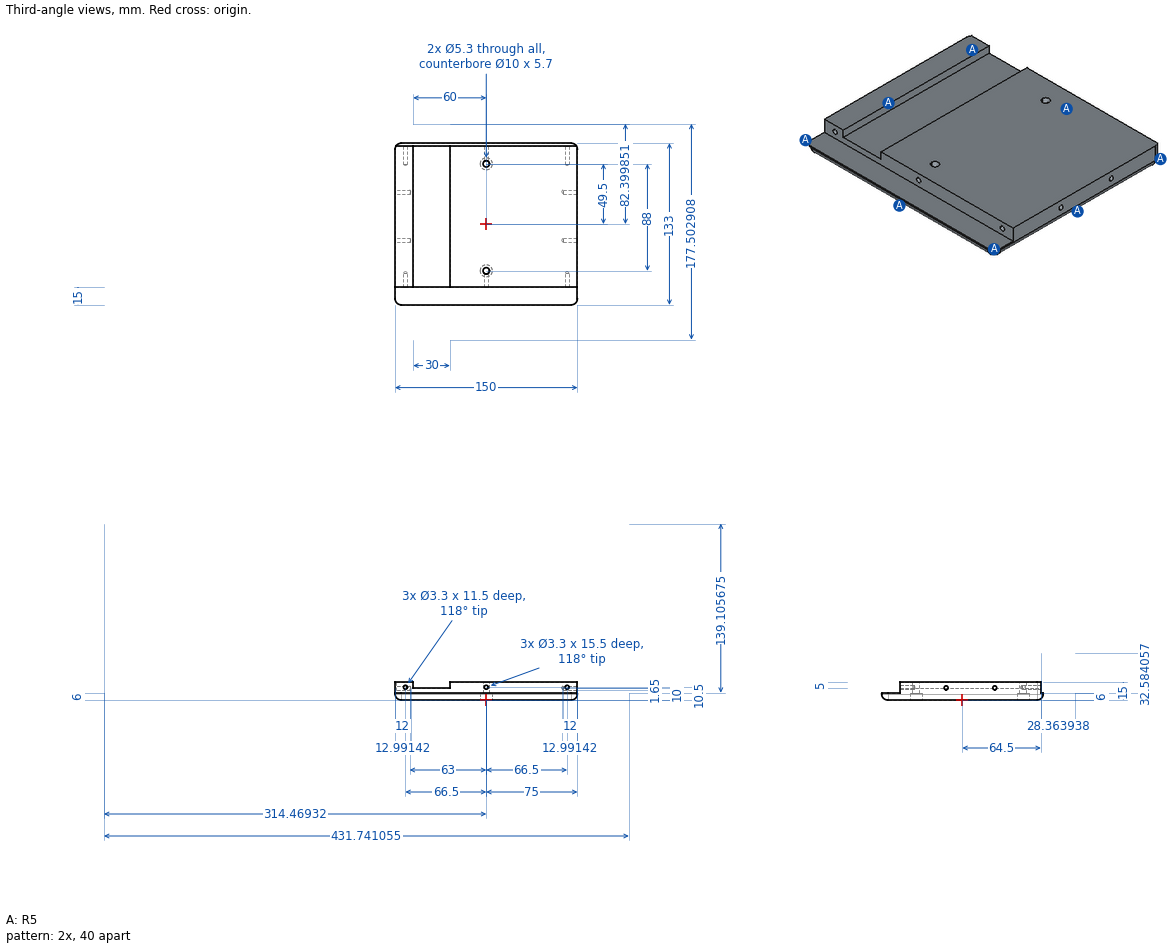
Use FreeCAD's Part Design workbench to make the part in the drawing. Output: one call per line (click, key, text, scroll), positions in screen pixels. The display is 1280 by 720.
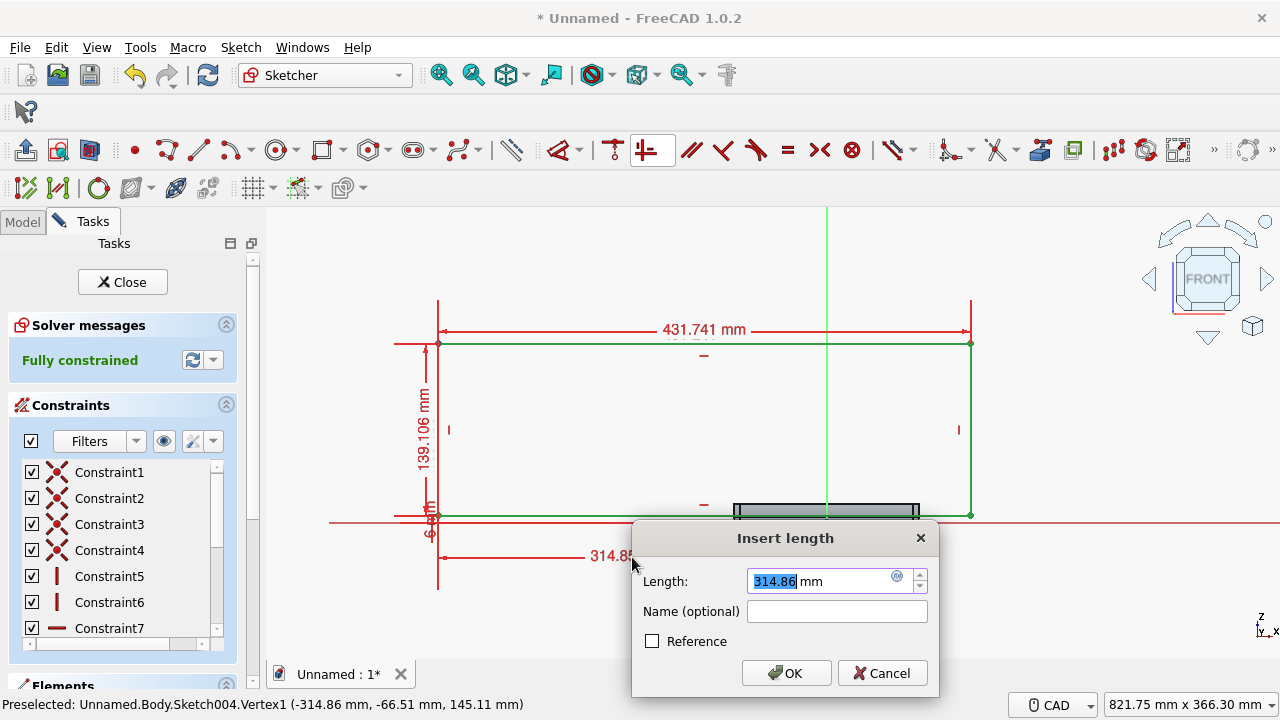
text(314.46932)
key(Return)
key(Escape)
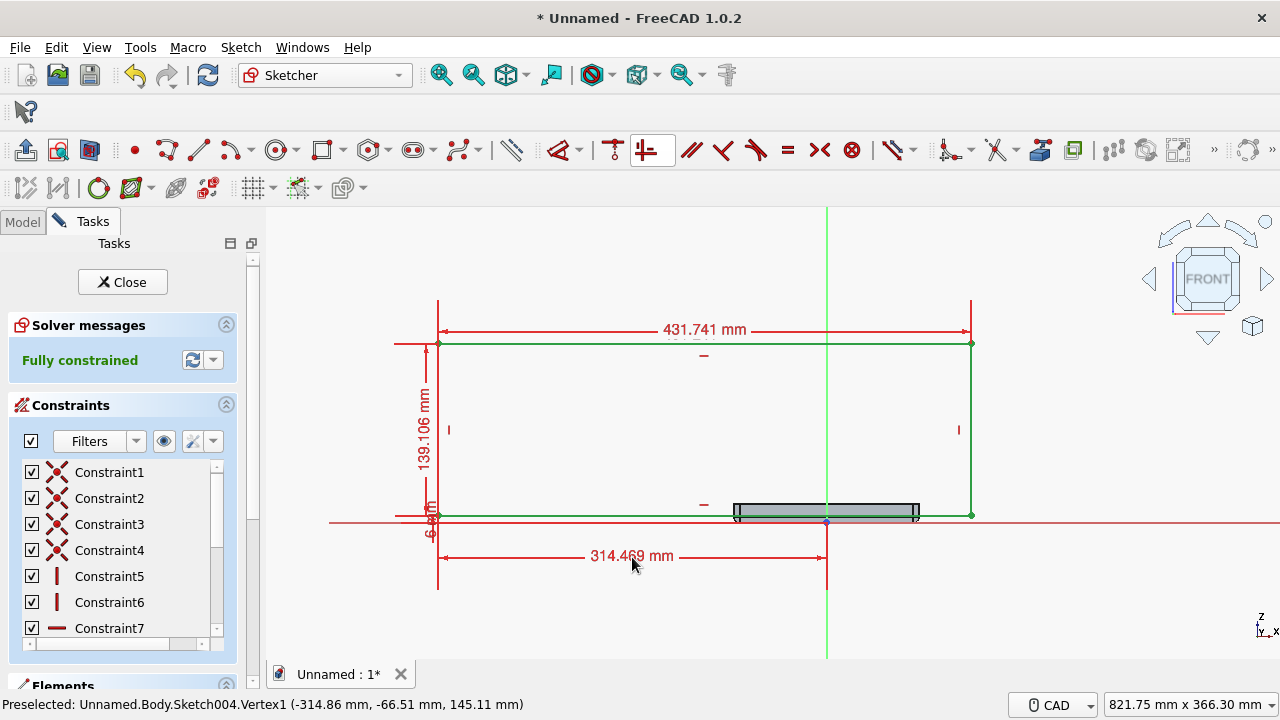
click(123, 282)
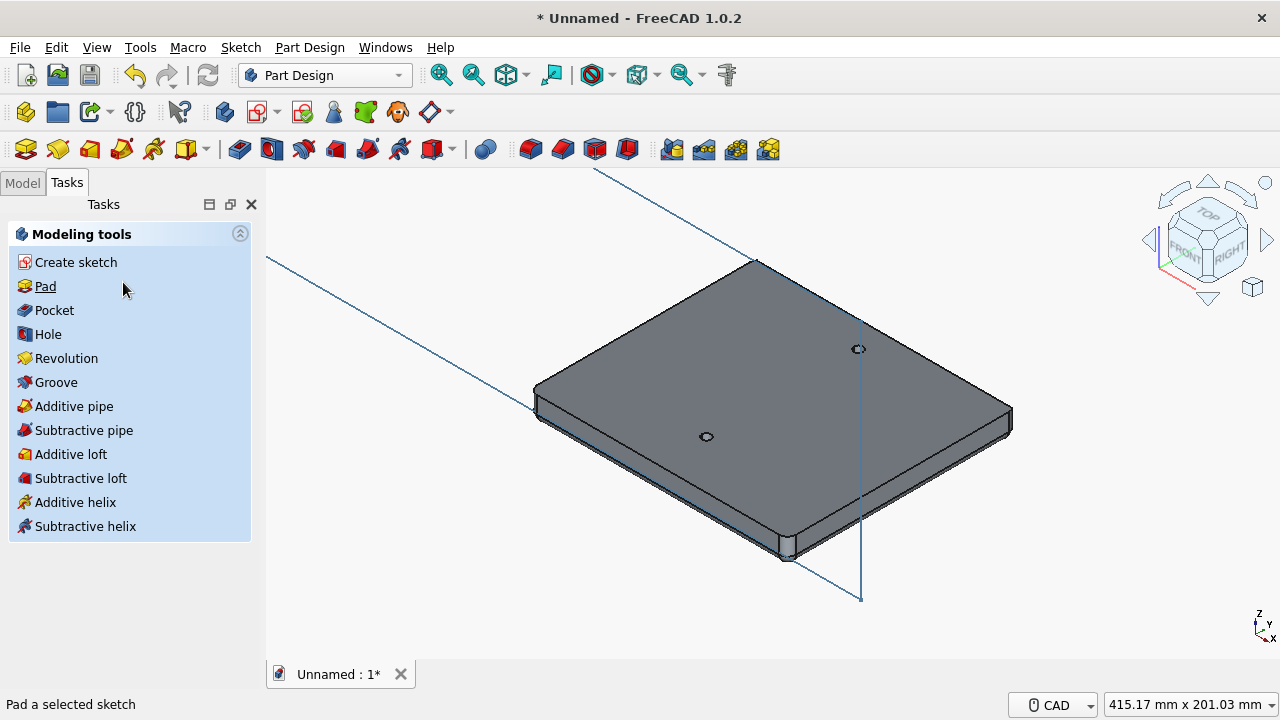
click(240, 150)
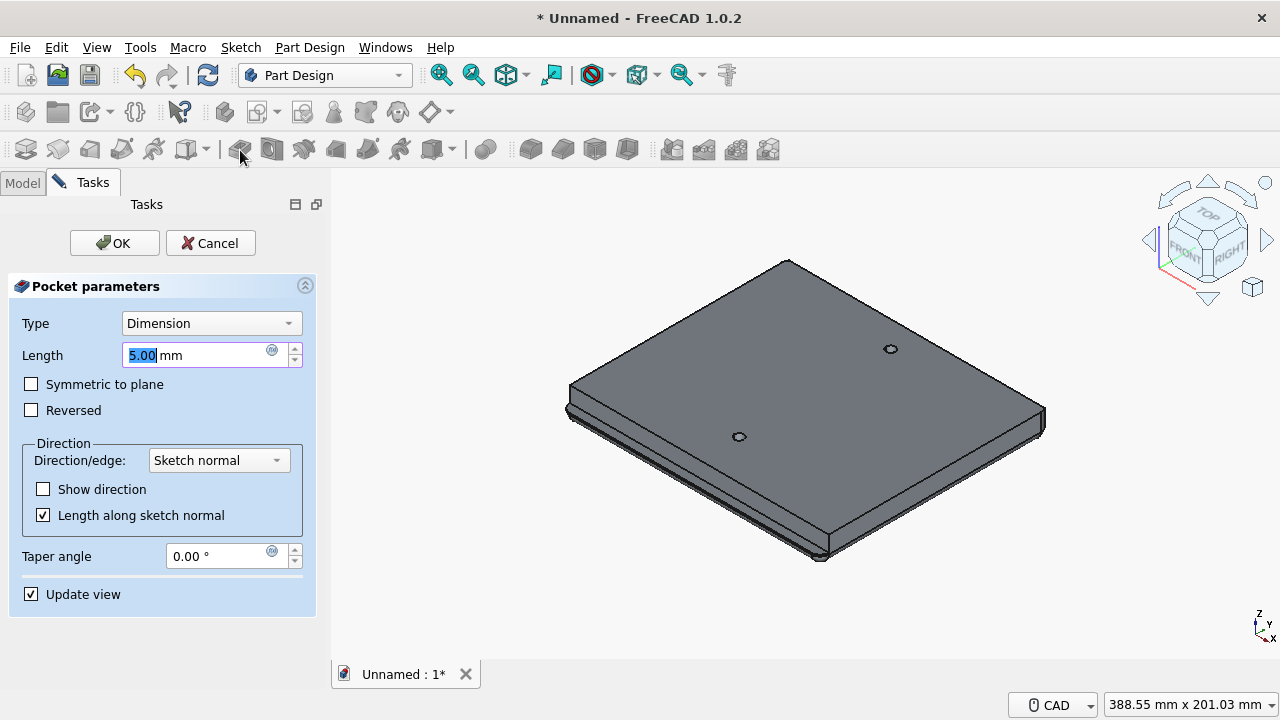
text(15)
key(Tab)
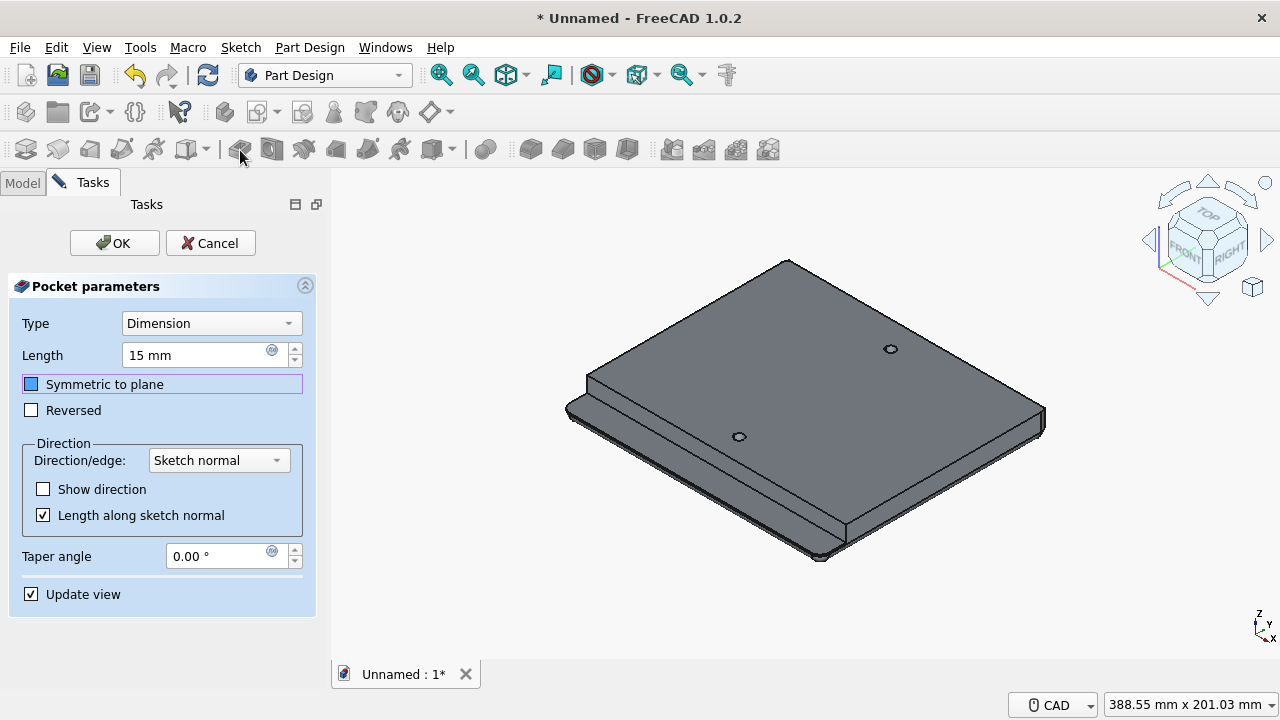
click(115, 243)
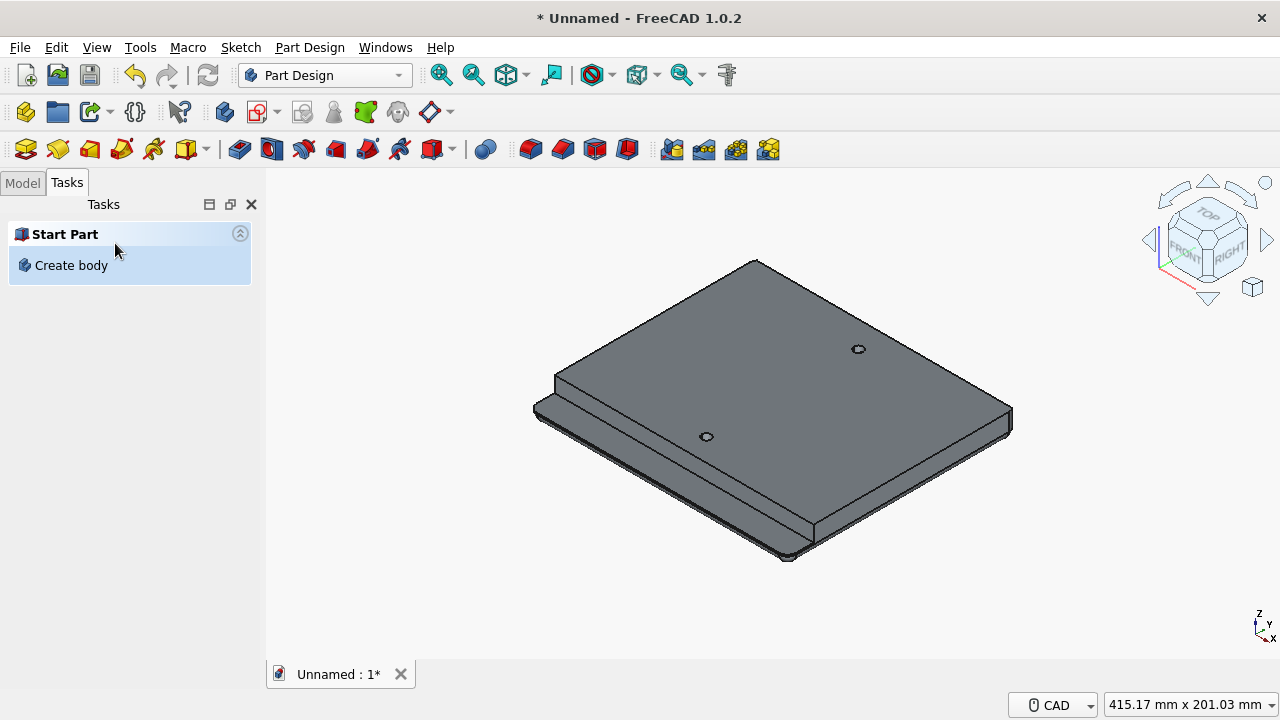
click(821, 412)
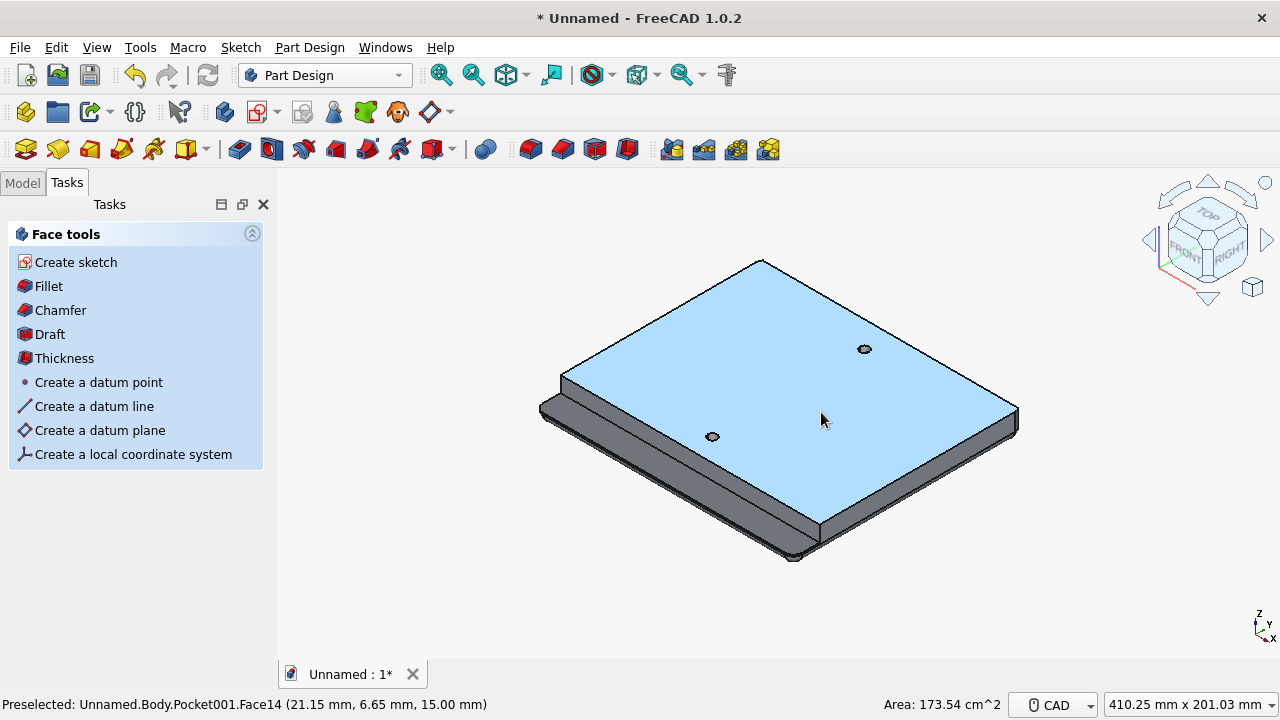
click(258, 112)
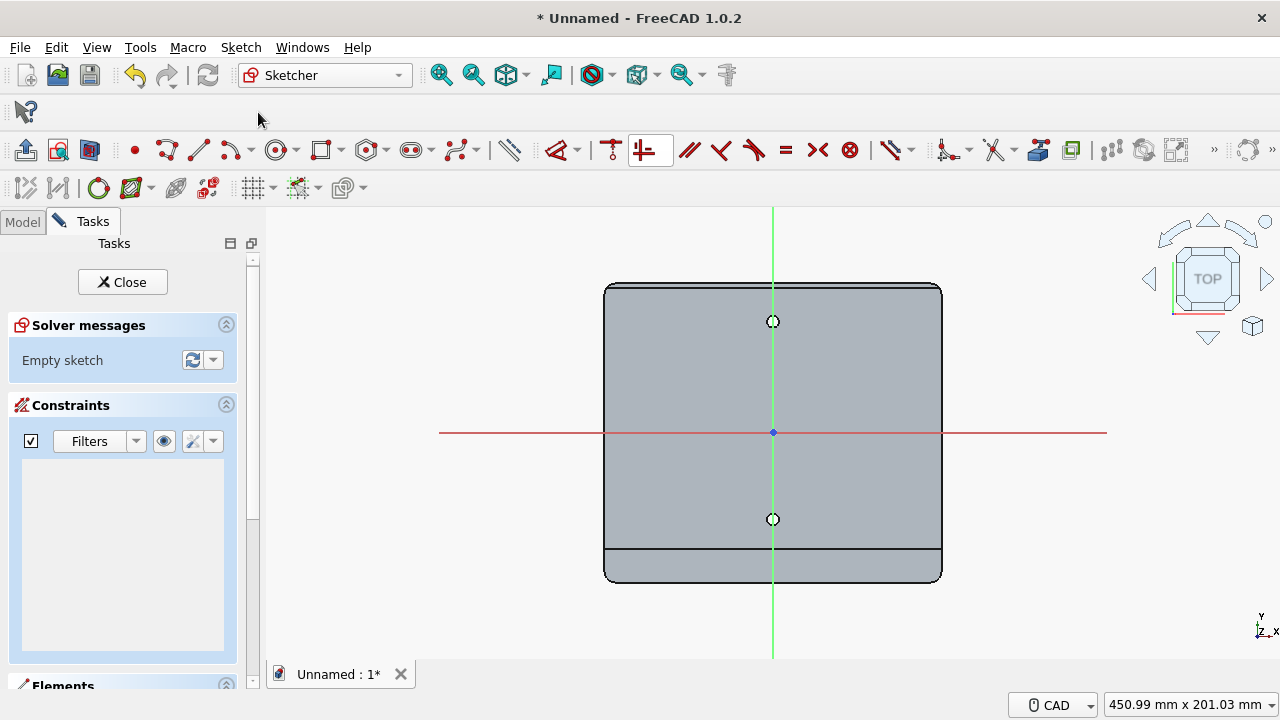
scroll(702, 404, down, 2)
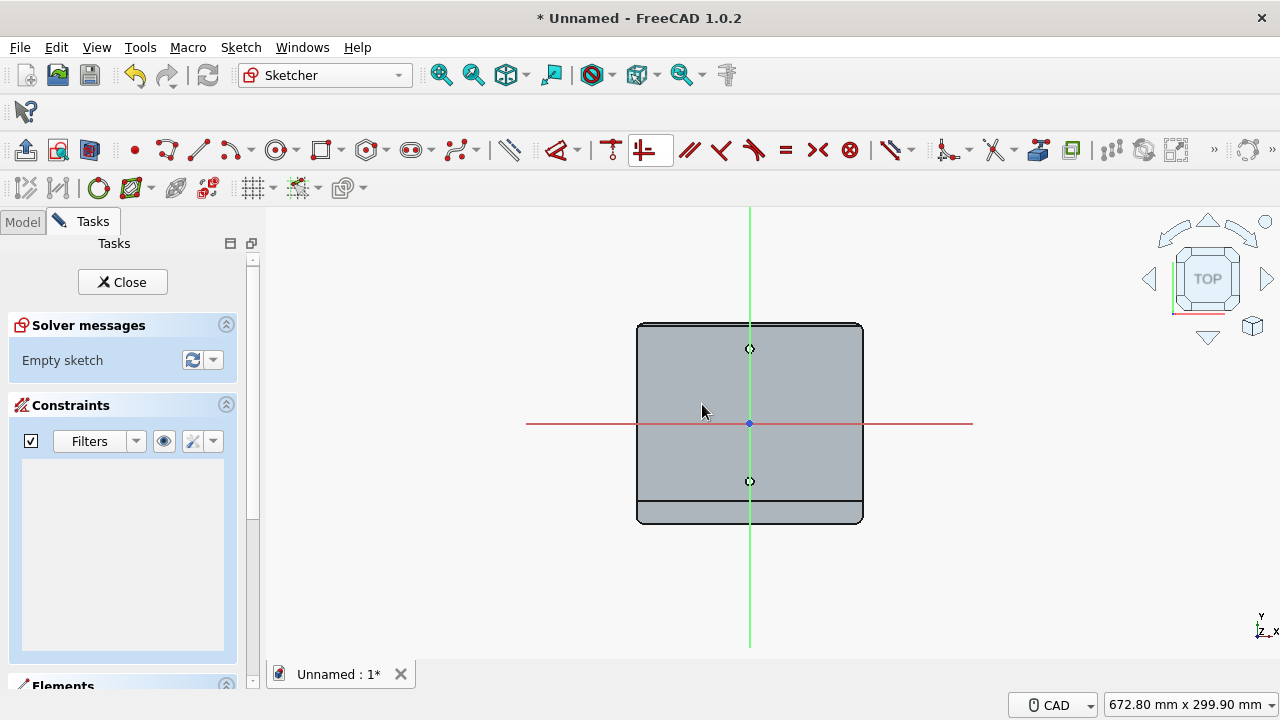
click(322, 150)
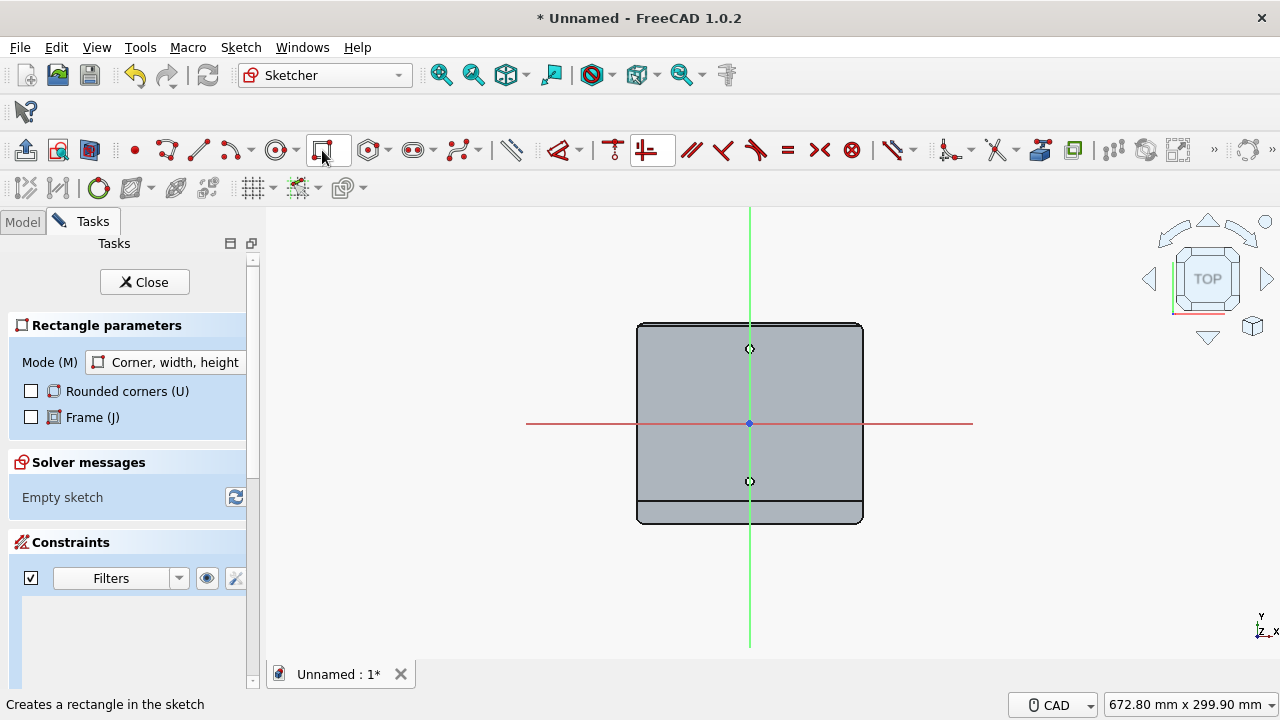
click(659, 299)
move(705, 567)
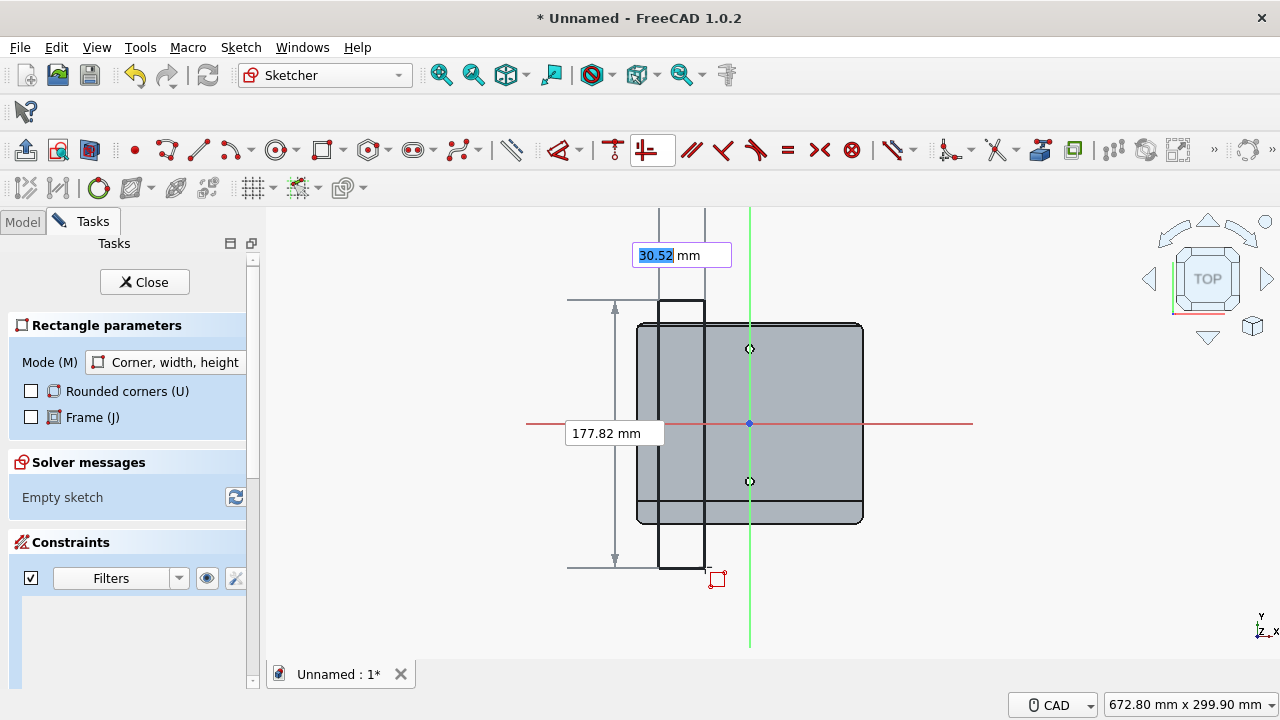
text(30)
key(Tab)
text(177.502908)
key(Return)
key(Escape)